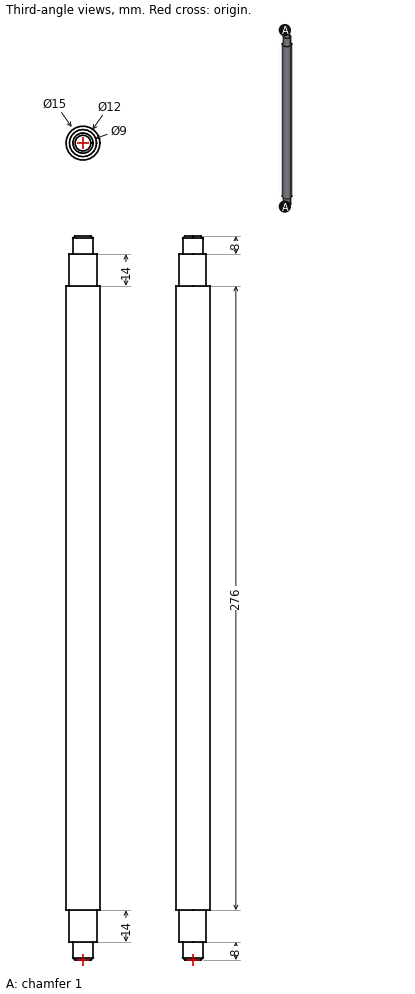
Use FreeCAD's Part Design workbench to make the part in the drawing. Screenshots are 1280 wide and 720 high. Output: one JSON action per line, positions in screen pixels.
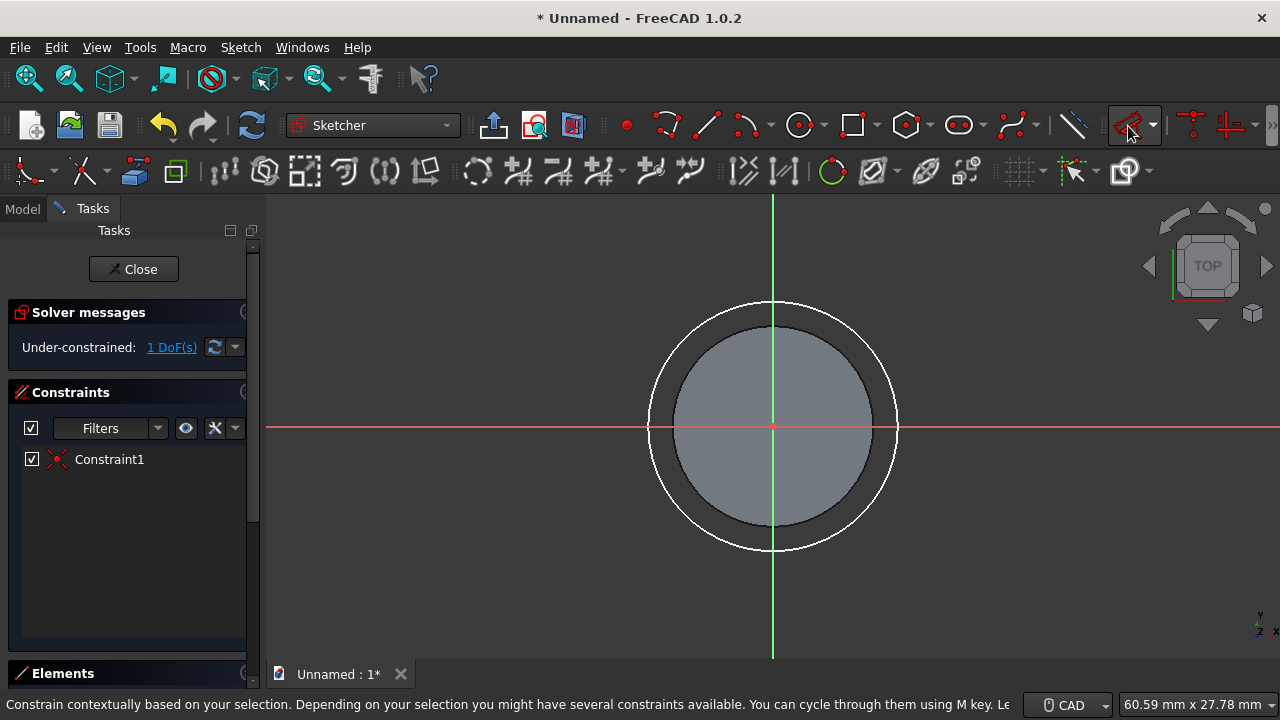
{"action": "left_click", "coordinate": [861, 338]}
{"action": "left_click", "coordinate": [884, 315]}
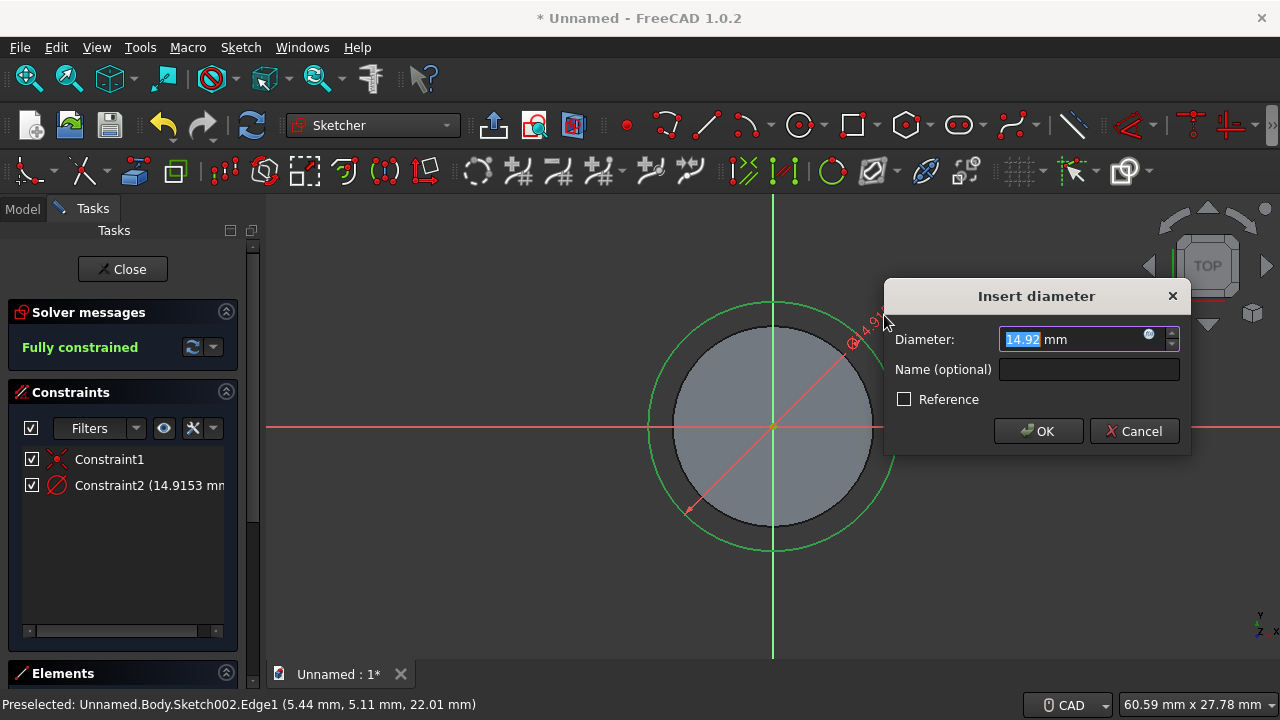
{"action": "type", "text": "15"}
{"action": "key", "text": "Return"}
{"action": "key", "text": "Escape"}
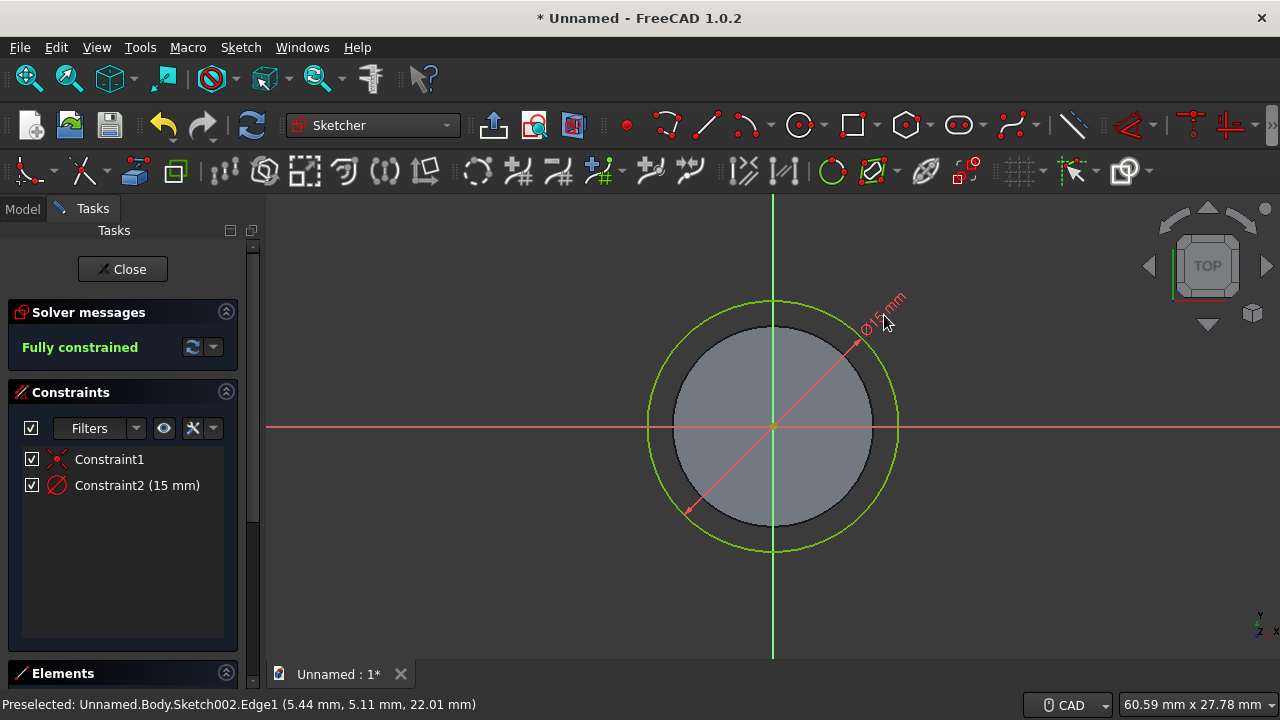
{"action": "left_click", "coordinate": [123, 269]}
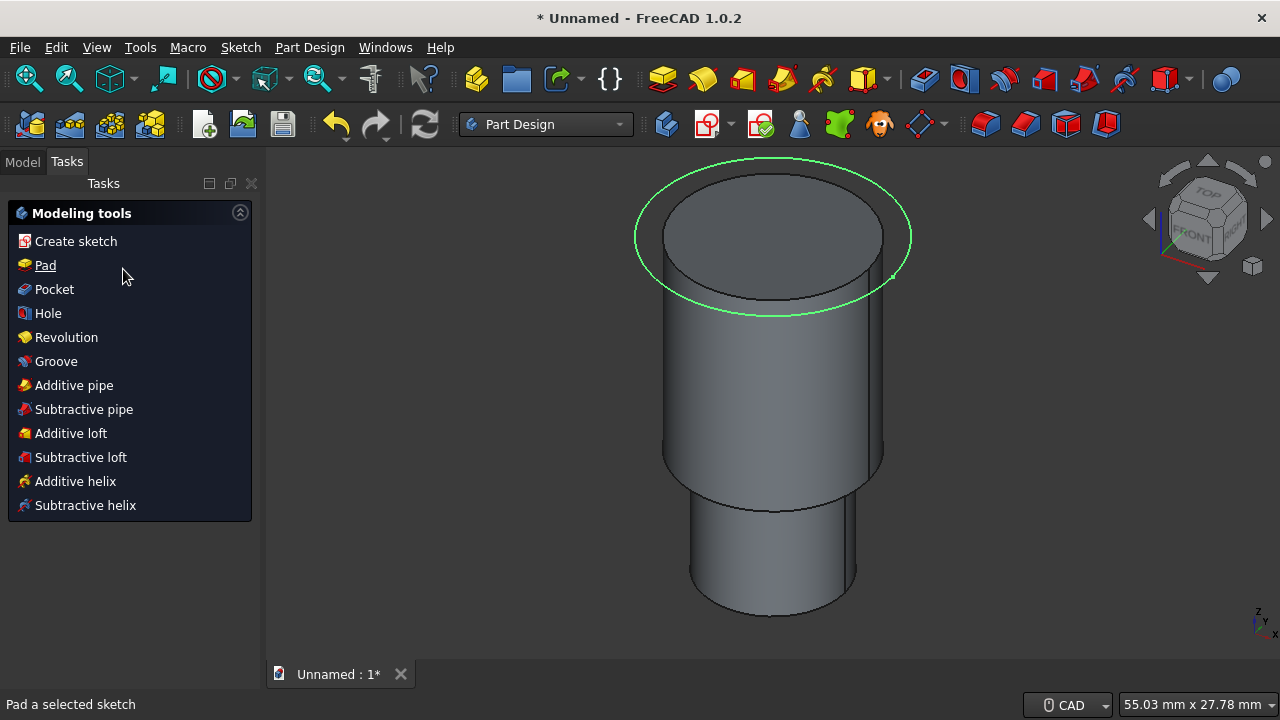
{"action": "left_click", "coordinate": [664, 80]}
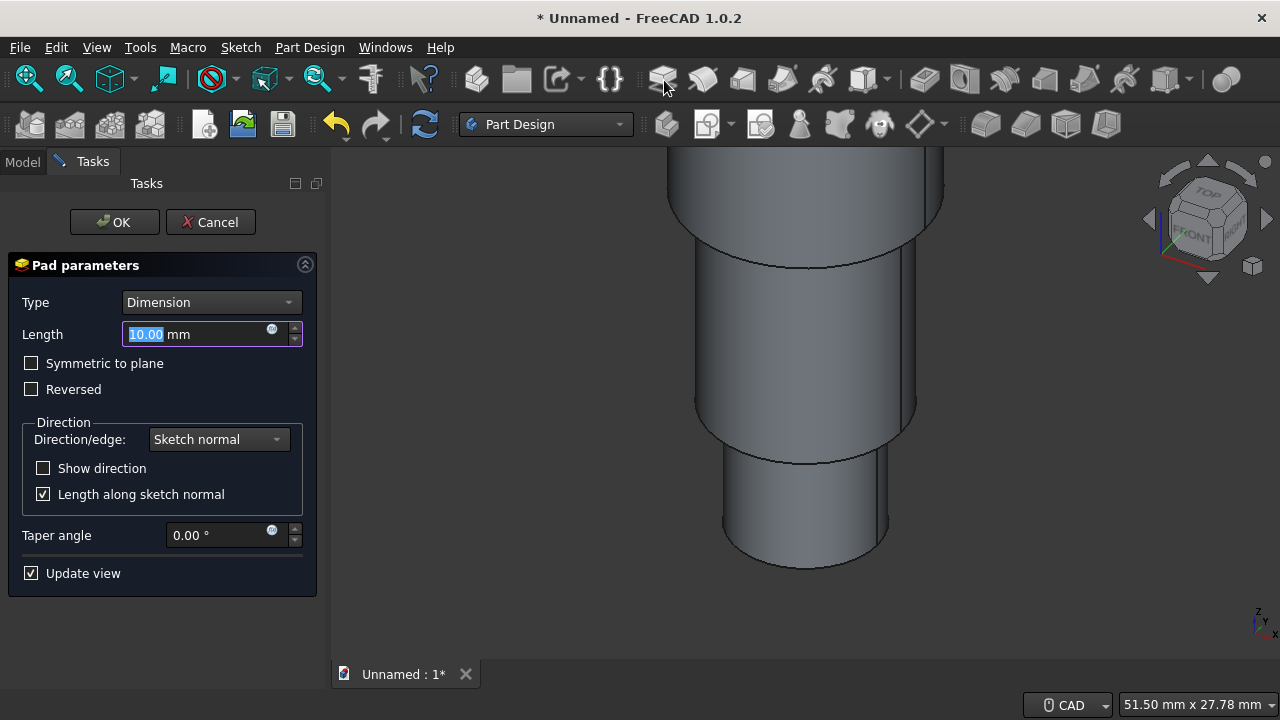
{"action": "type", "text": "276"}
{"action": "key", "text": "Tab"}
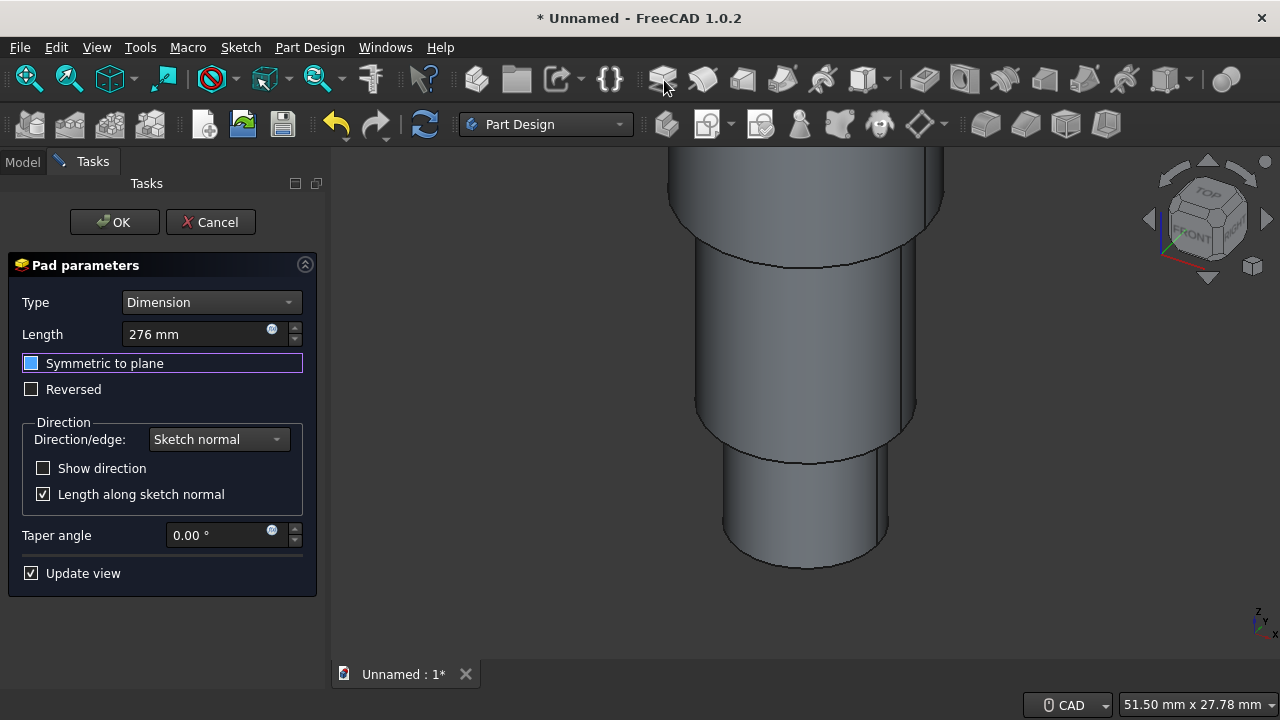
{"action": "left_click", "coordinate": [115, 222]}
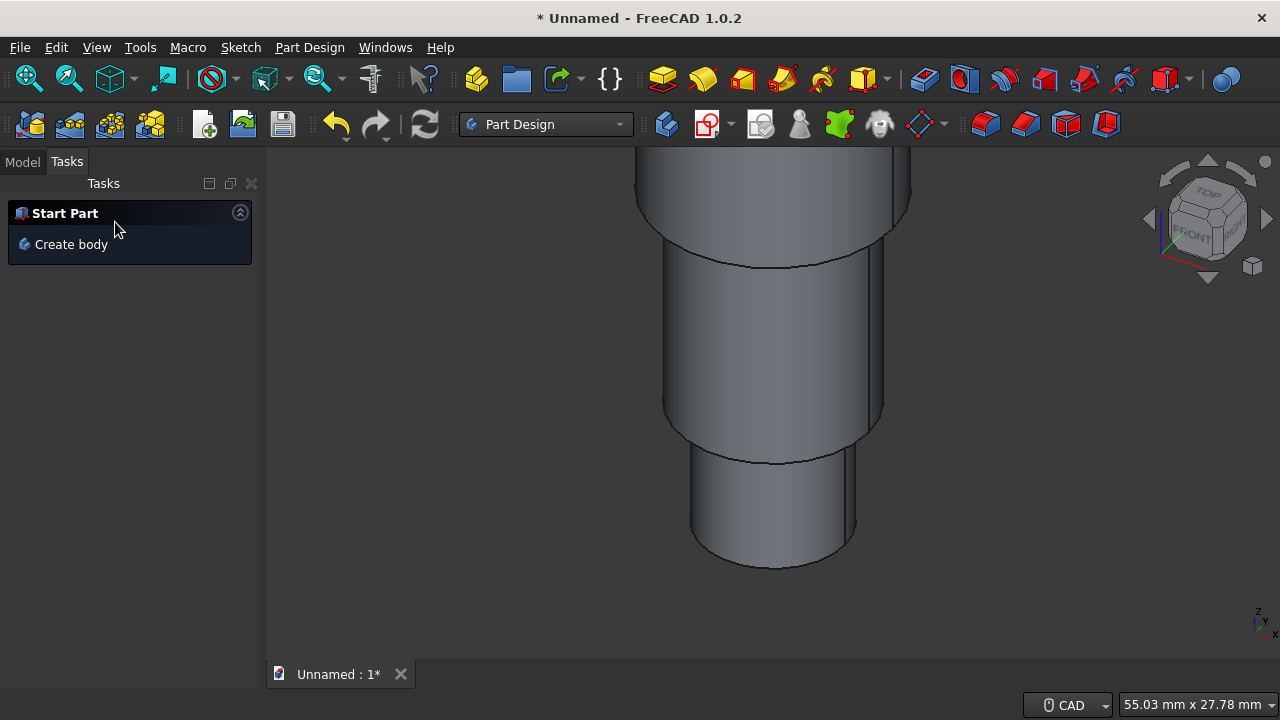
{"action": "key", "text": "v f"}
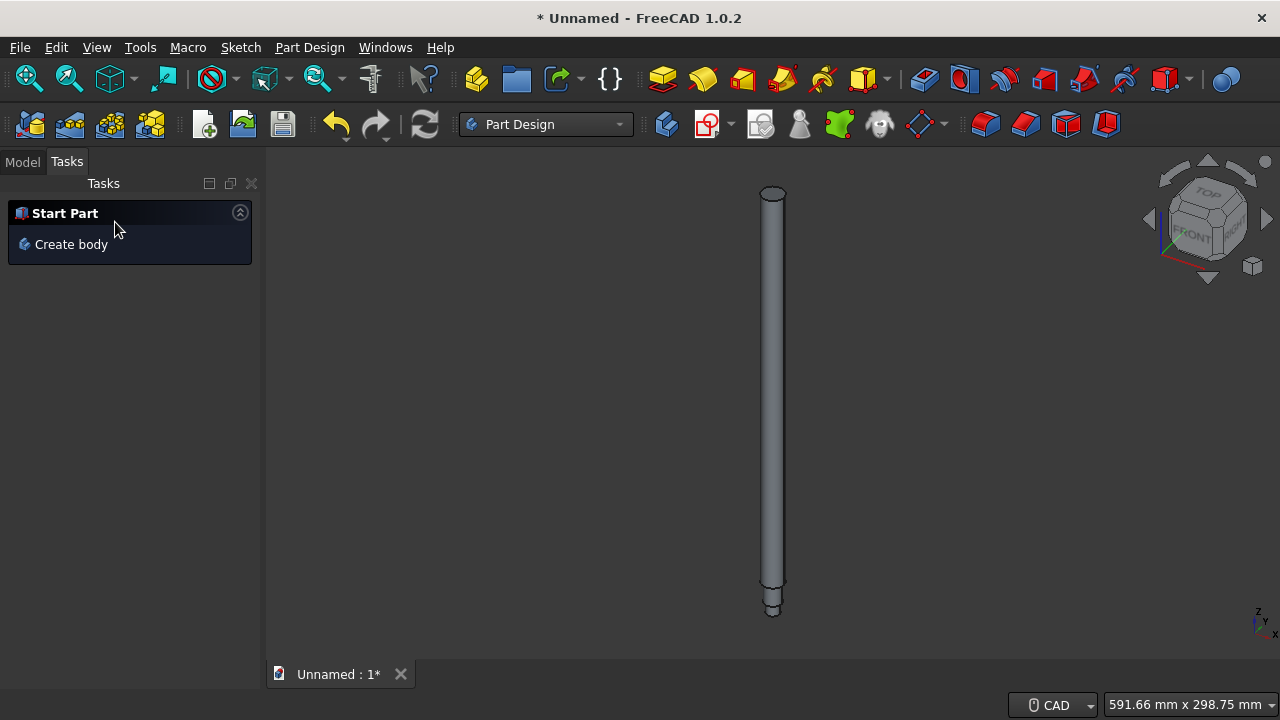
{"action": "left_click", "coordinate": [775, 191]}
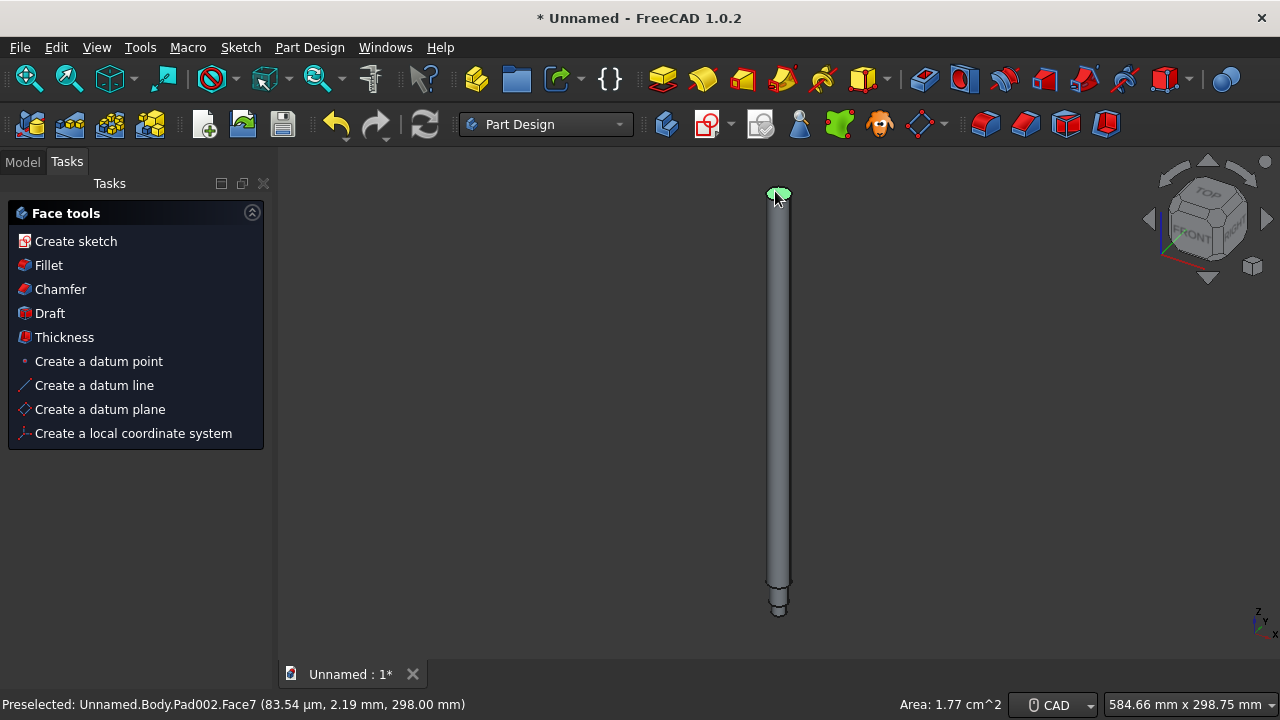
{"action": "left_click", "coordinate": [708, 124]}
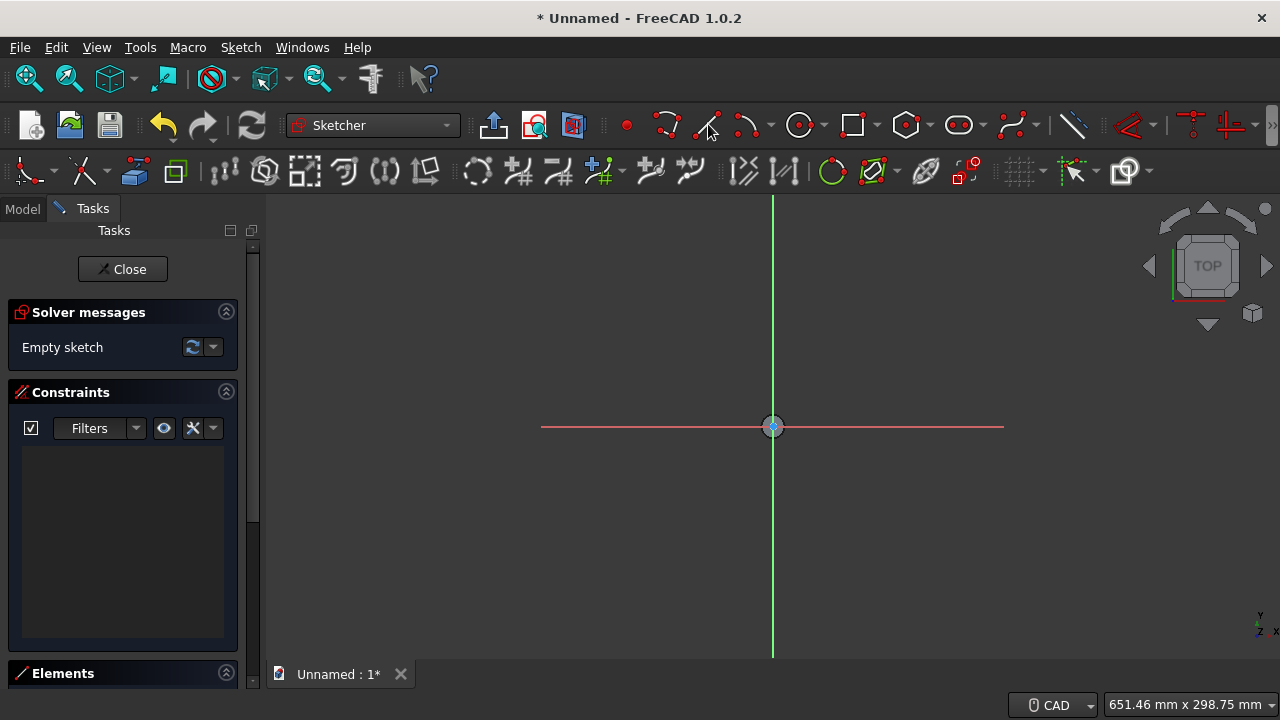
{"action": "scroll", "coordinate": [777, 426], "scroll_direction": "up", "scroll_amount": 14}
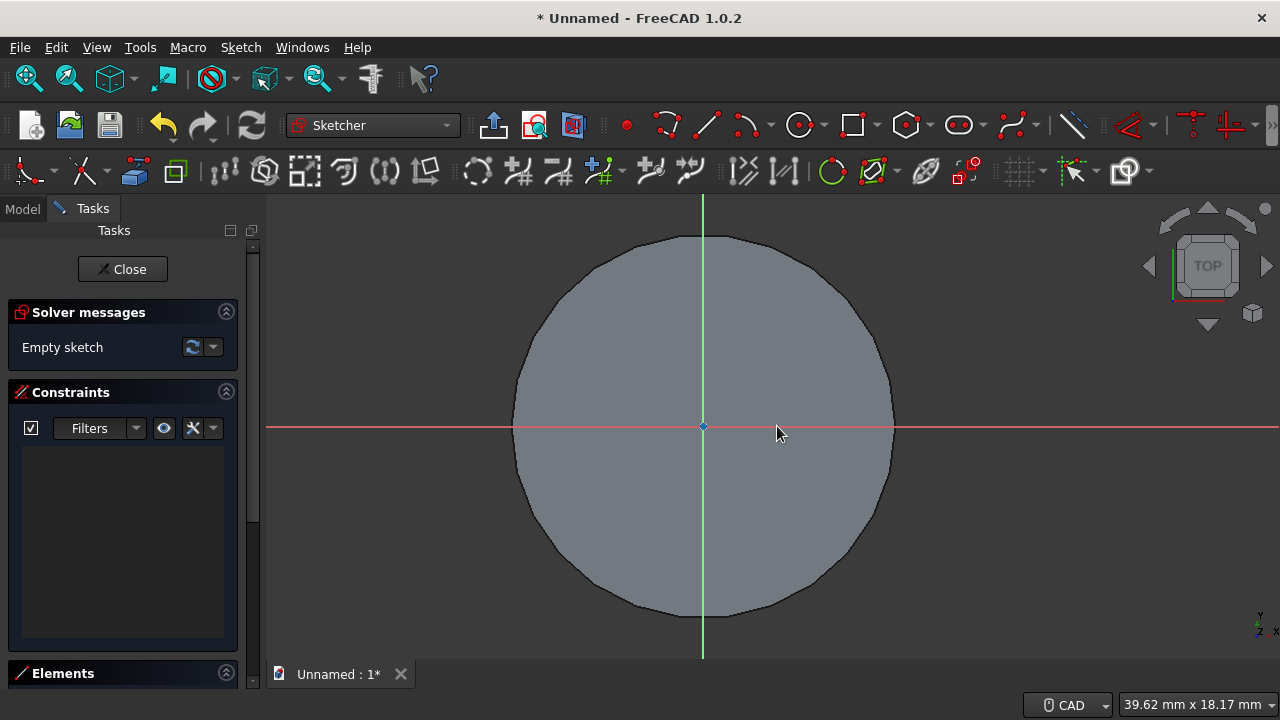
{"action": "key", "text": "g c"}